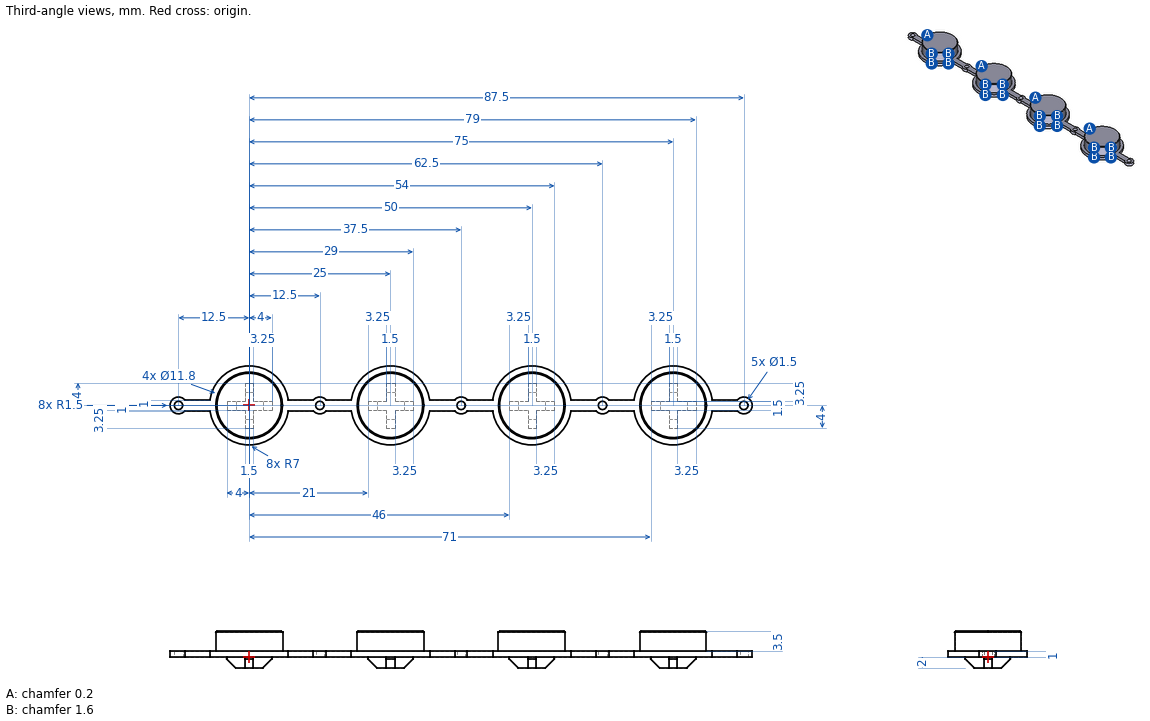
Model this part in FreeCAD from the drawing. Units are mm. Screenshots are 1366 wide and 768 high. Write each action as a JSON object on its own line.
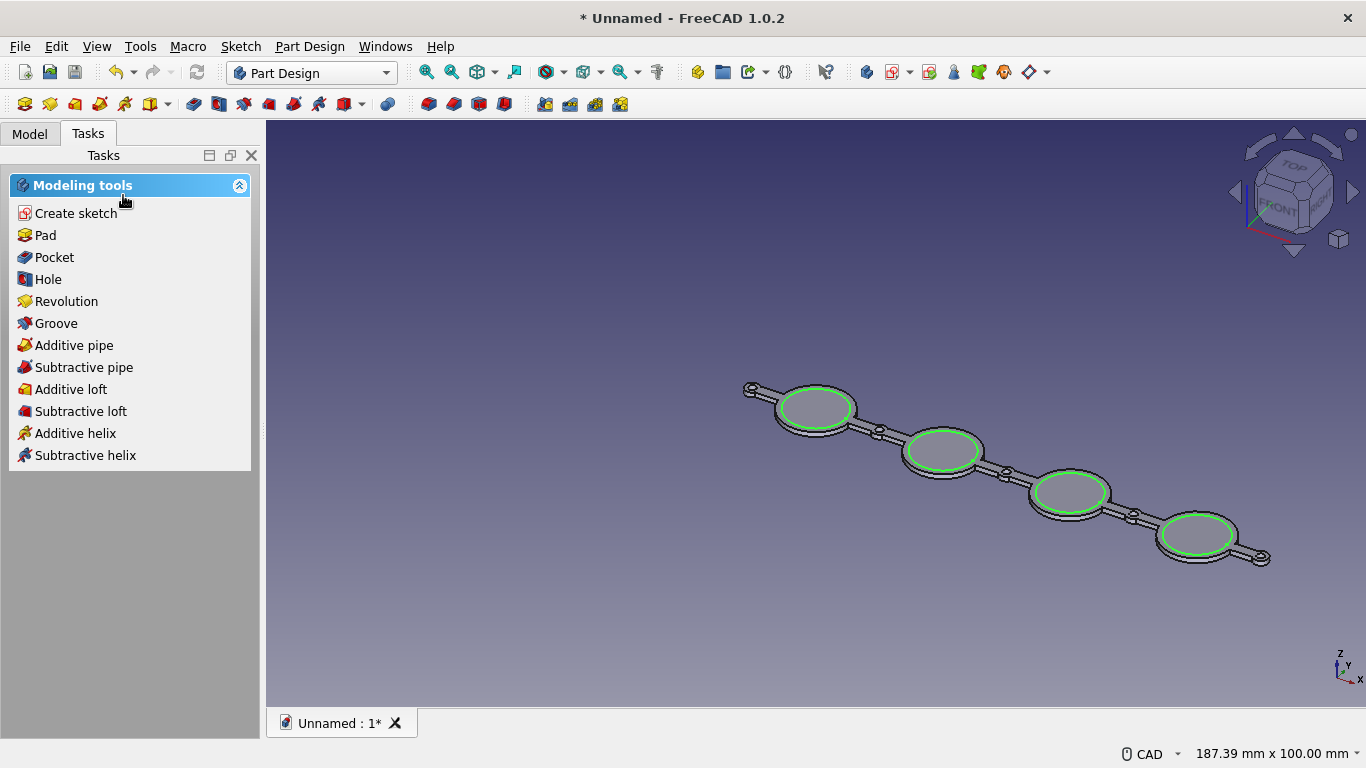
{"action": "left_click", "coordinate": [25, 104]}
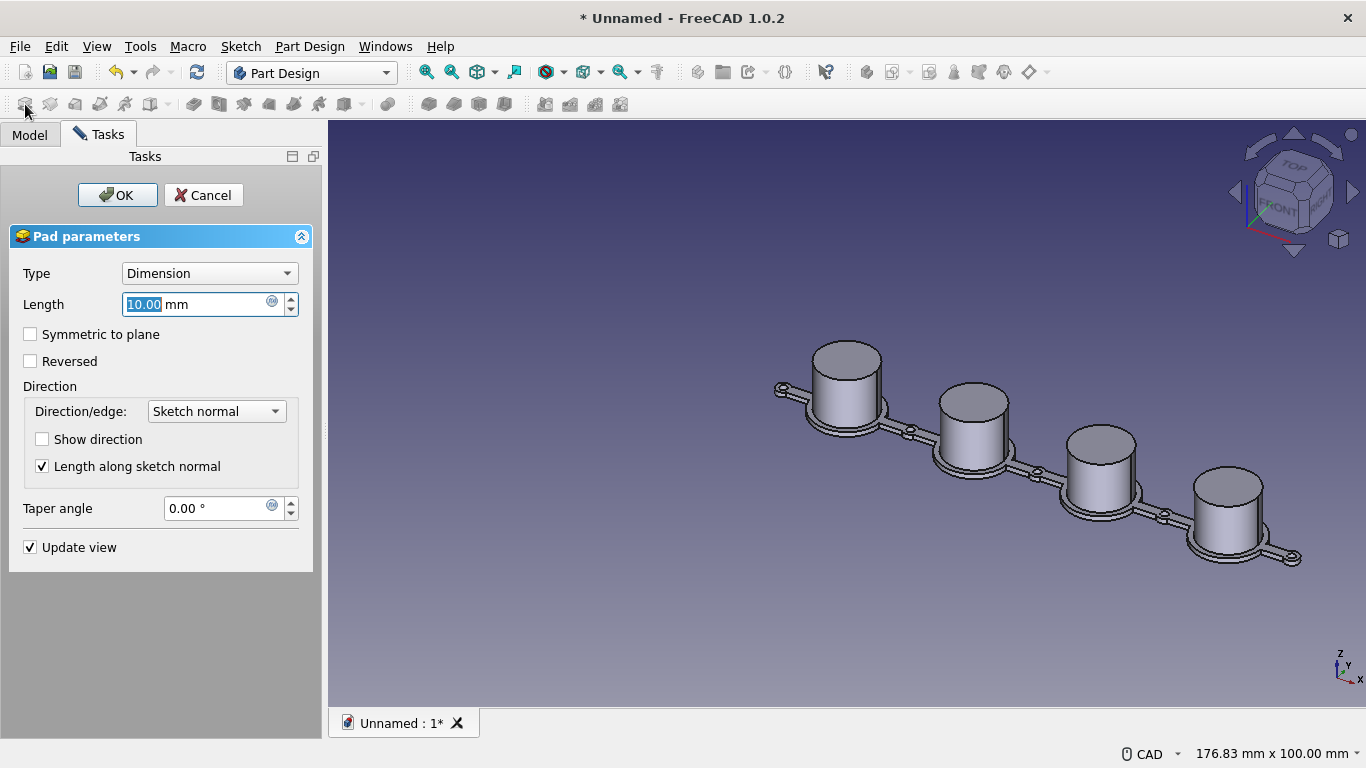
{"action": "type", "text": "3.5"}
{"action": "key", "text": "Tab"}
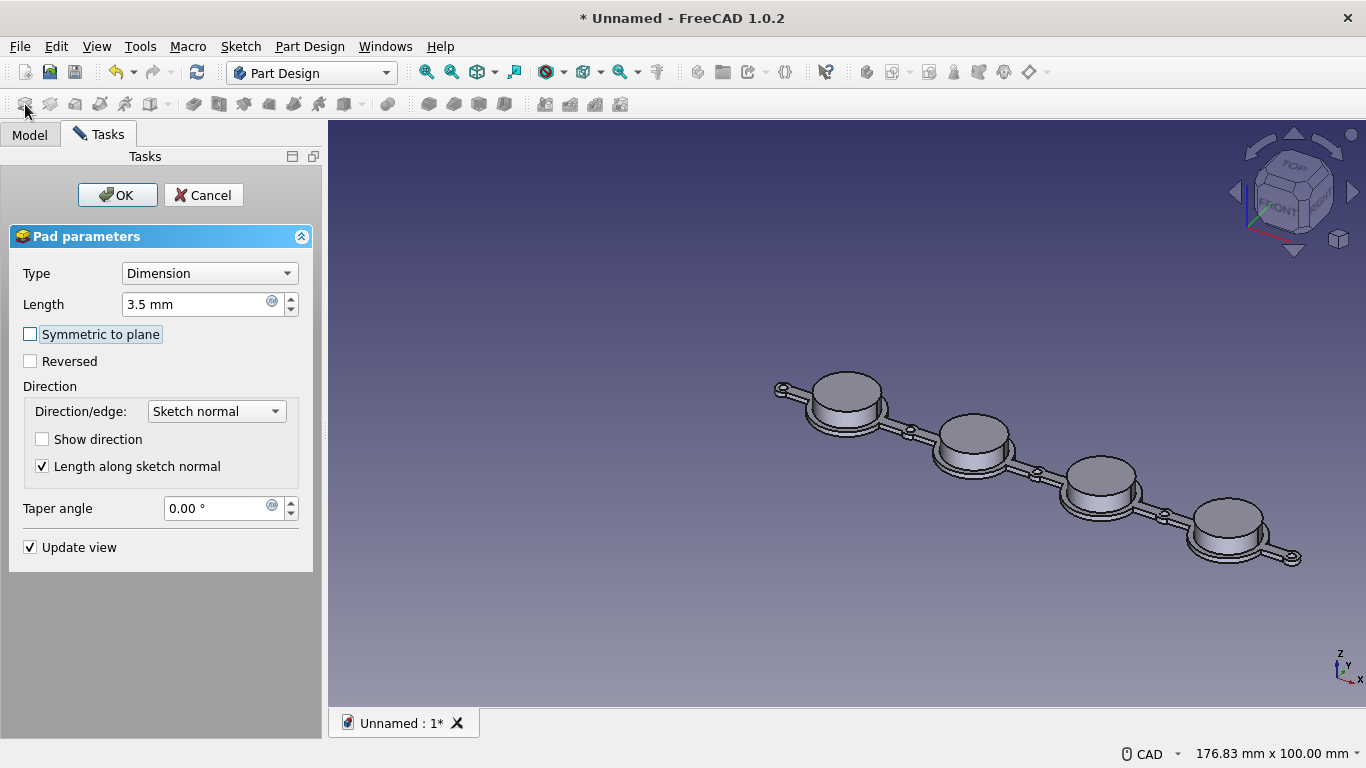
{"action": "left_click", "coordinate": [118, 195]}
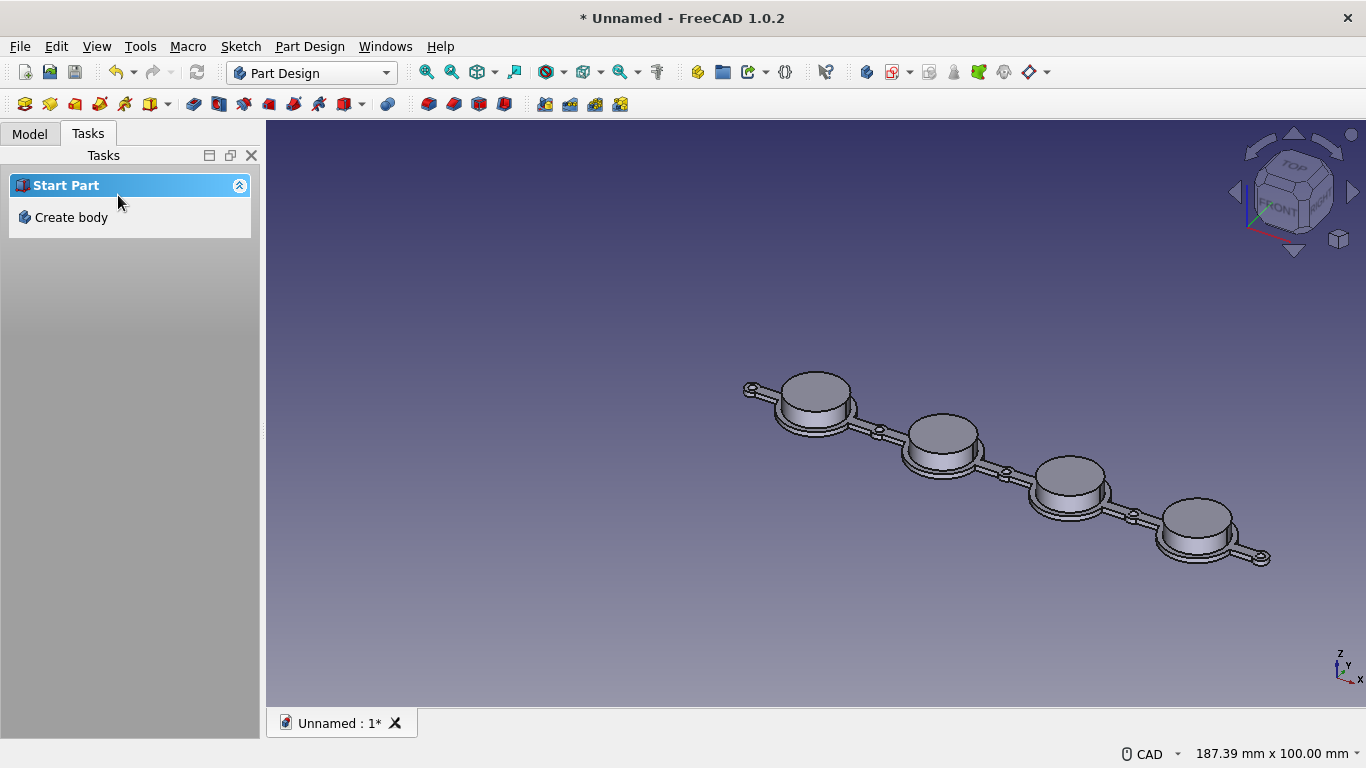
{"action": "left_click", "coordinate": [786, 381]}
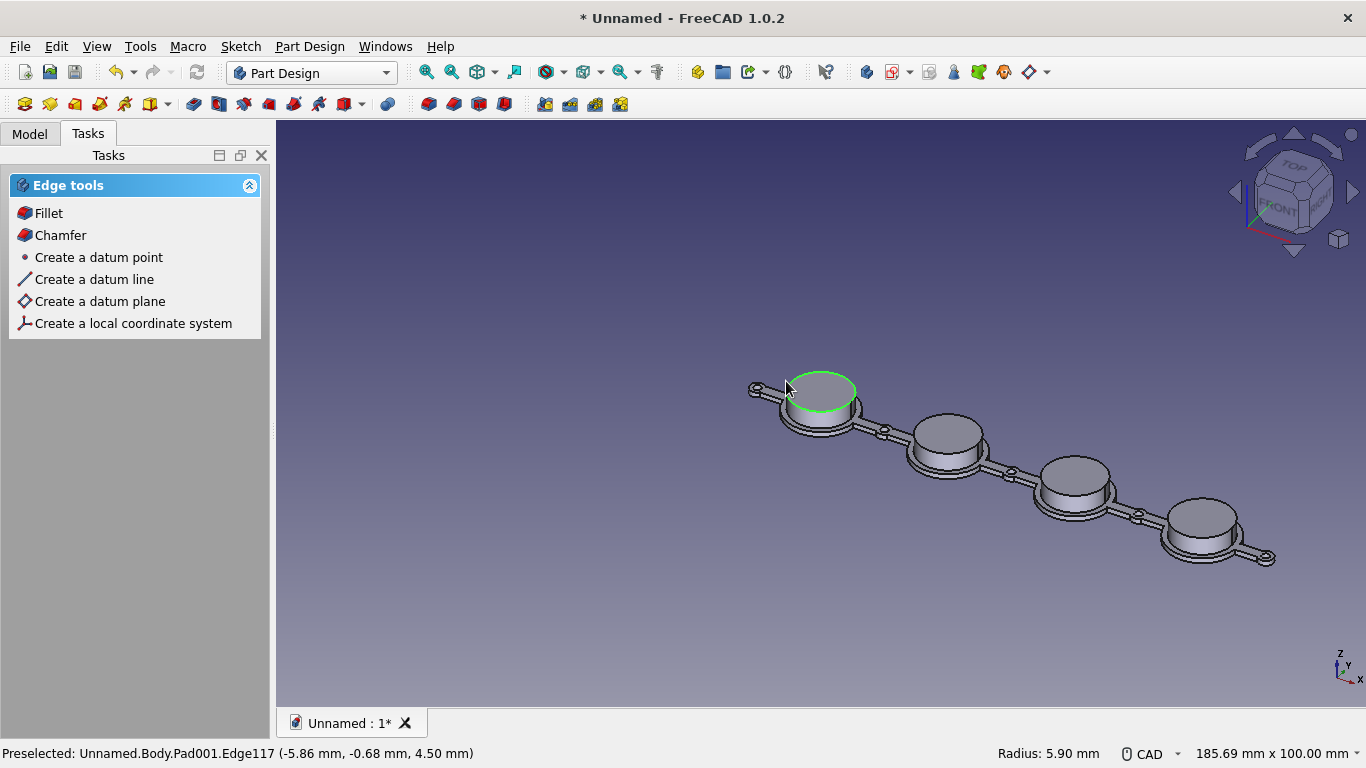
{"action": "left_click", "coordinate": [918, 423], "text": "ctrl"}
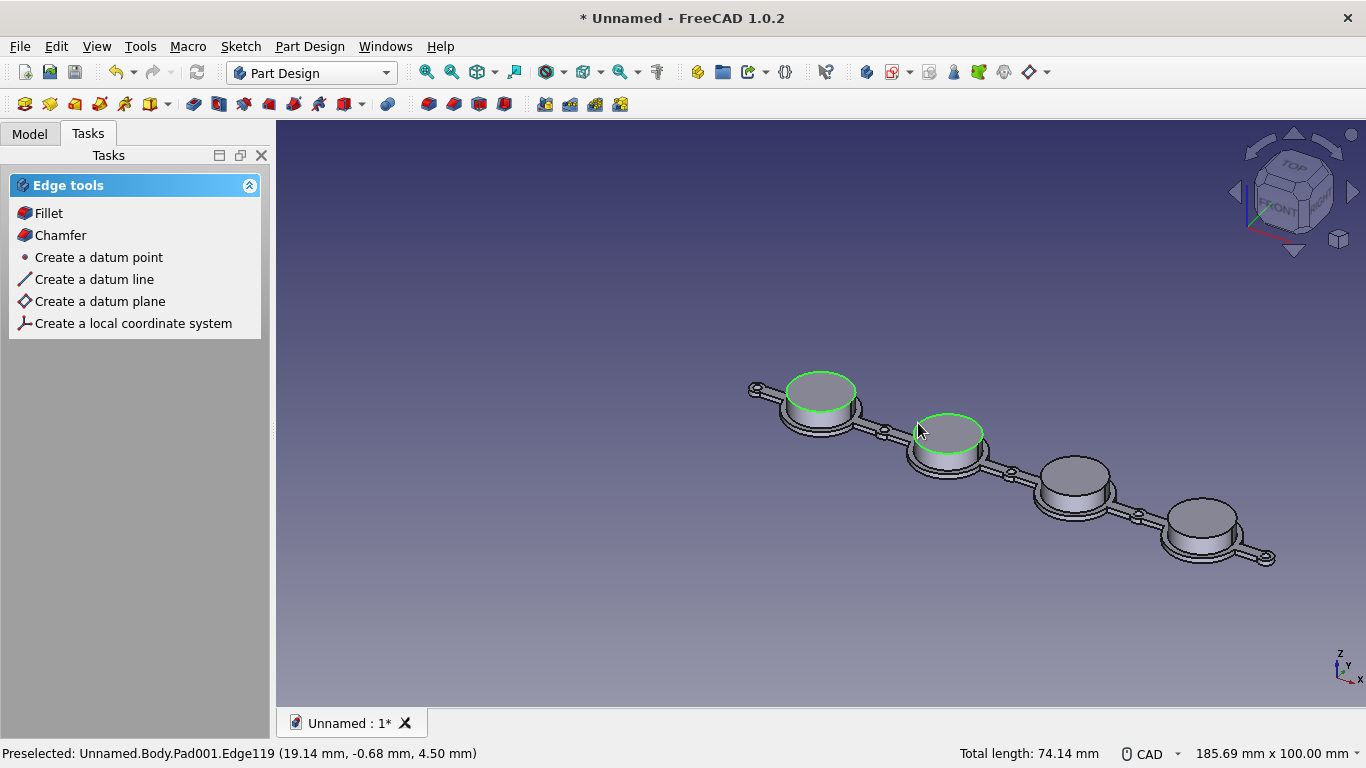
{"action": "left_click", "coordinate": [1045, 465], "text": "ctrl"}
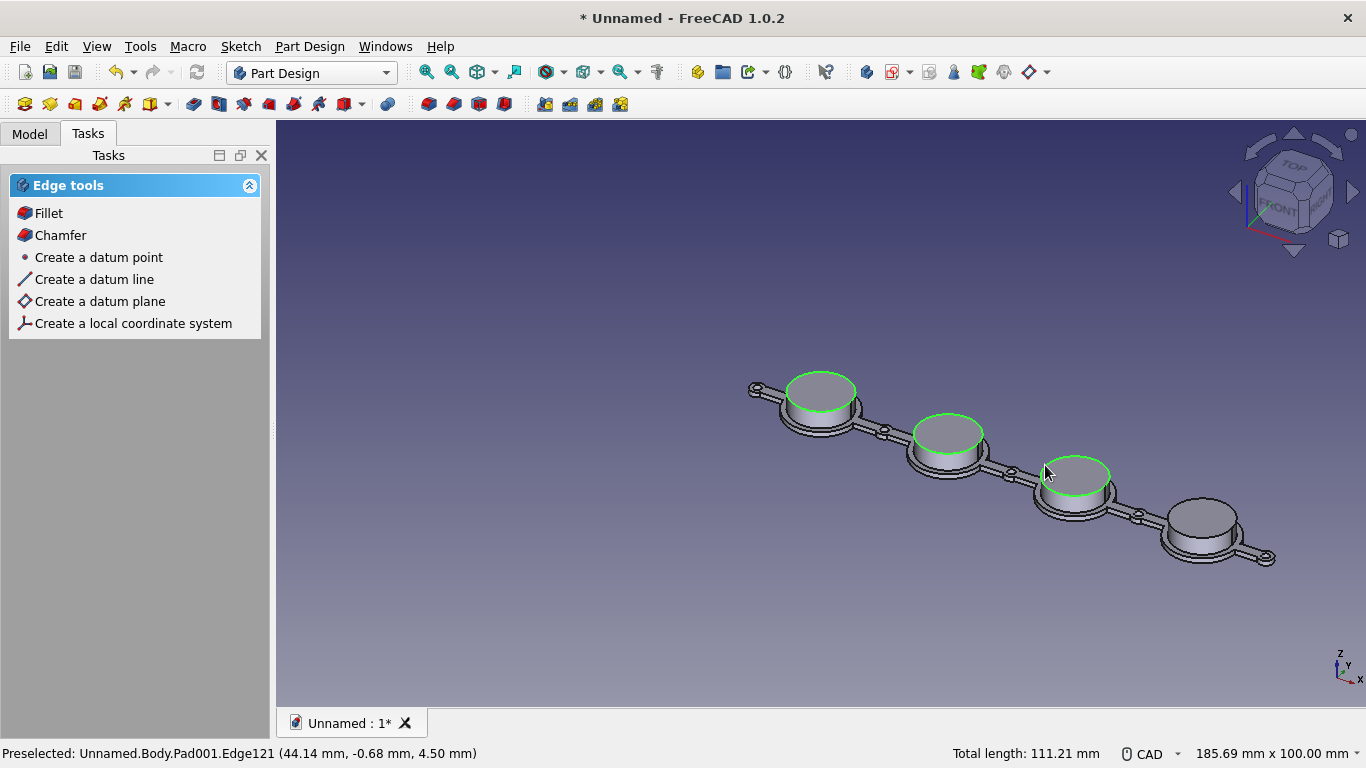
{"action": "left_click", "coordinate": [1172, 507], "text": "ctrl"}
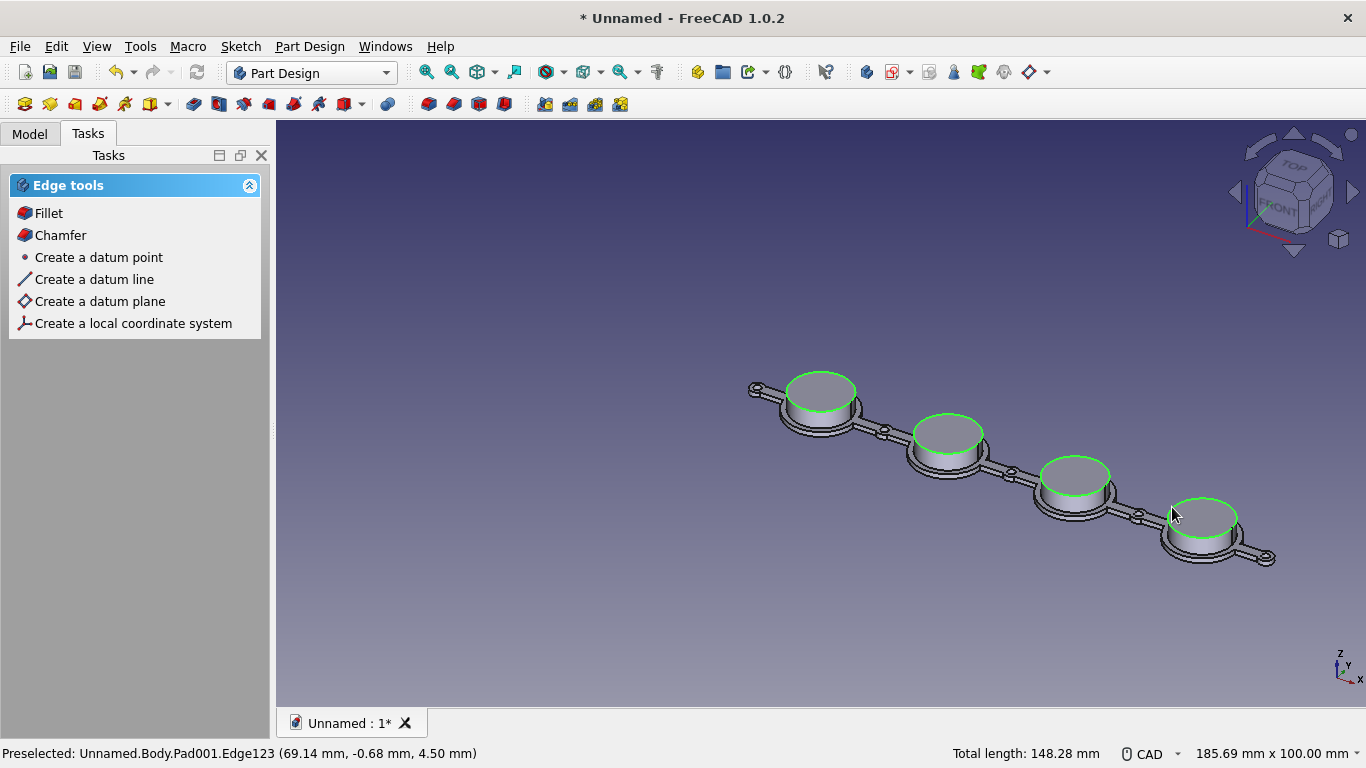
{"action": "left_click", "coordinate": [454, 104]}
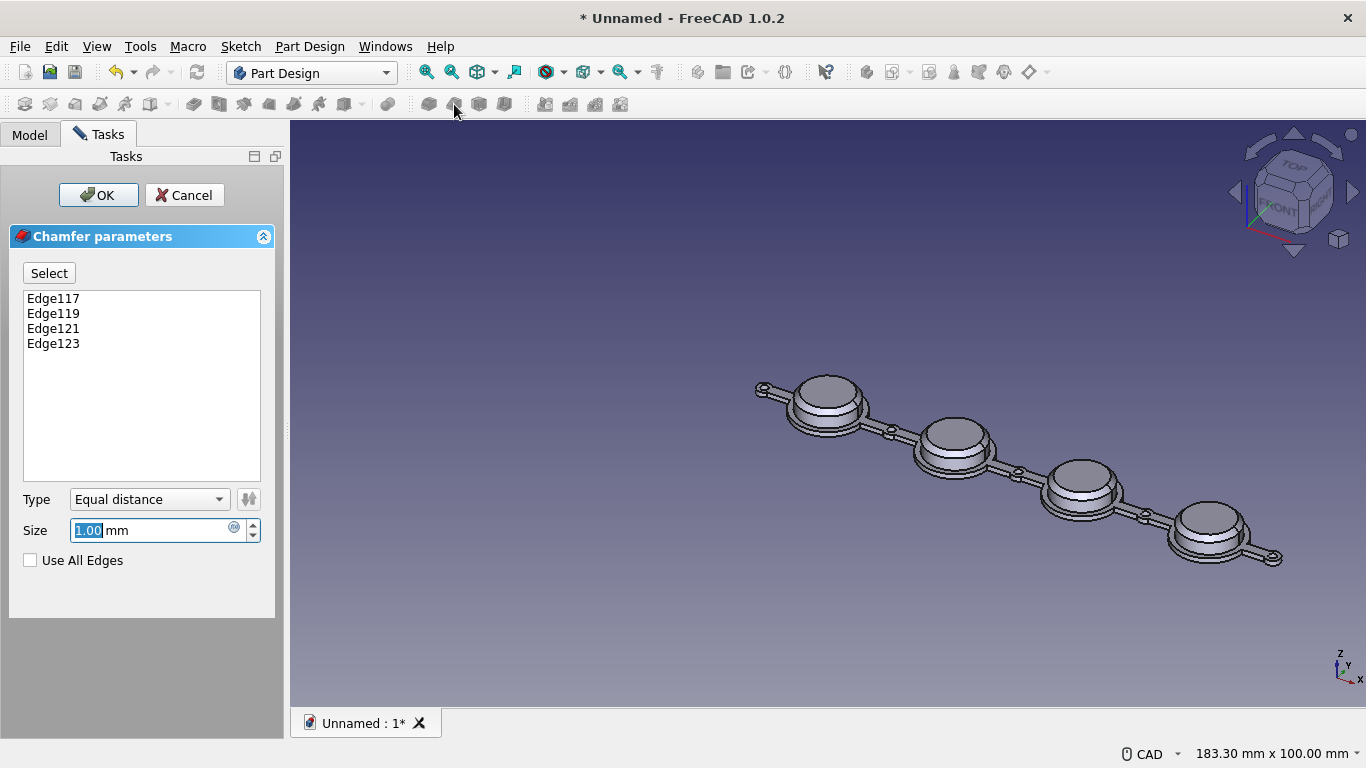
{"action": "type", "text": "0.2"}
{"action": "key", "text": "Tab"}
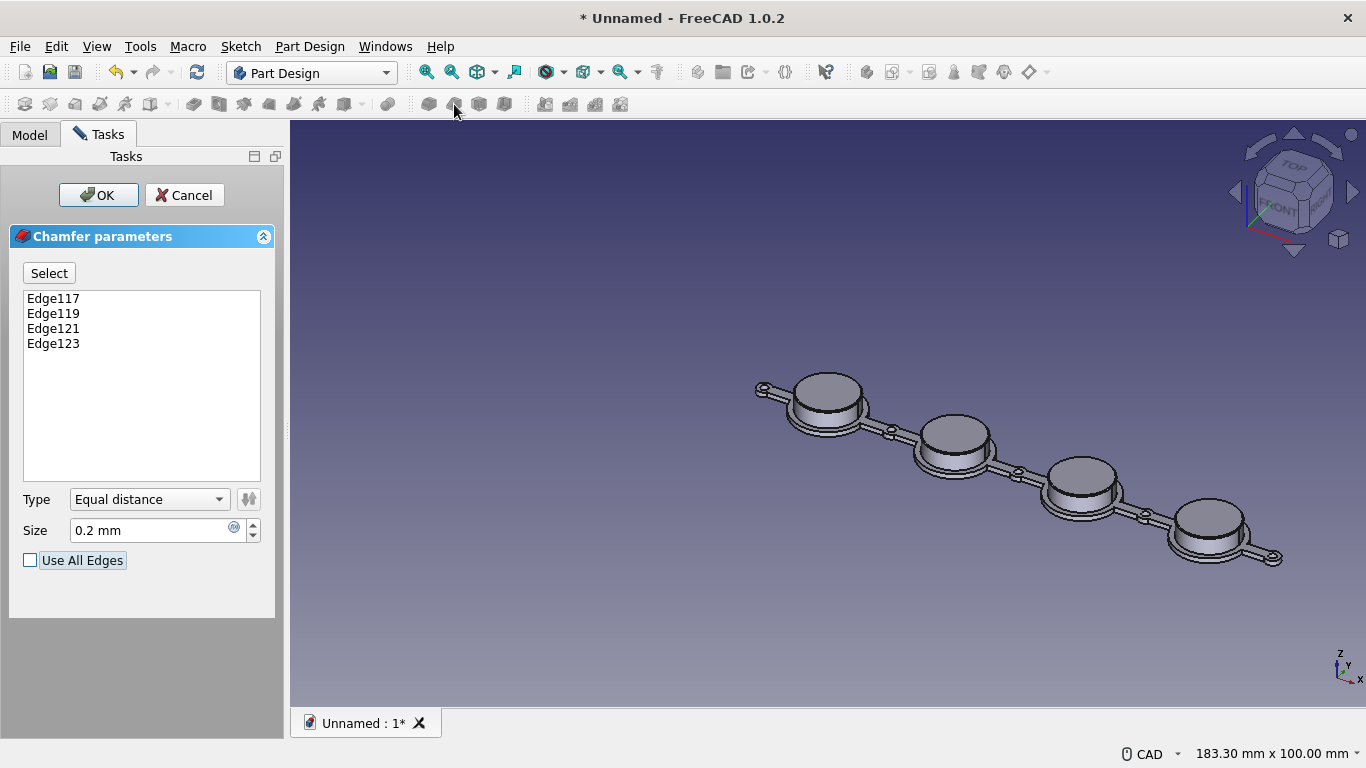
{"action": "left_click", "coordinate": [99, 195]}